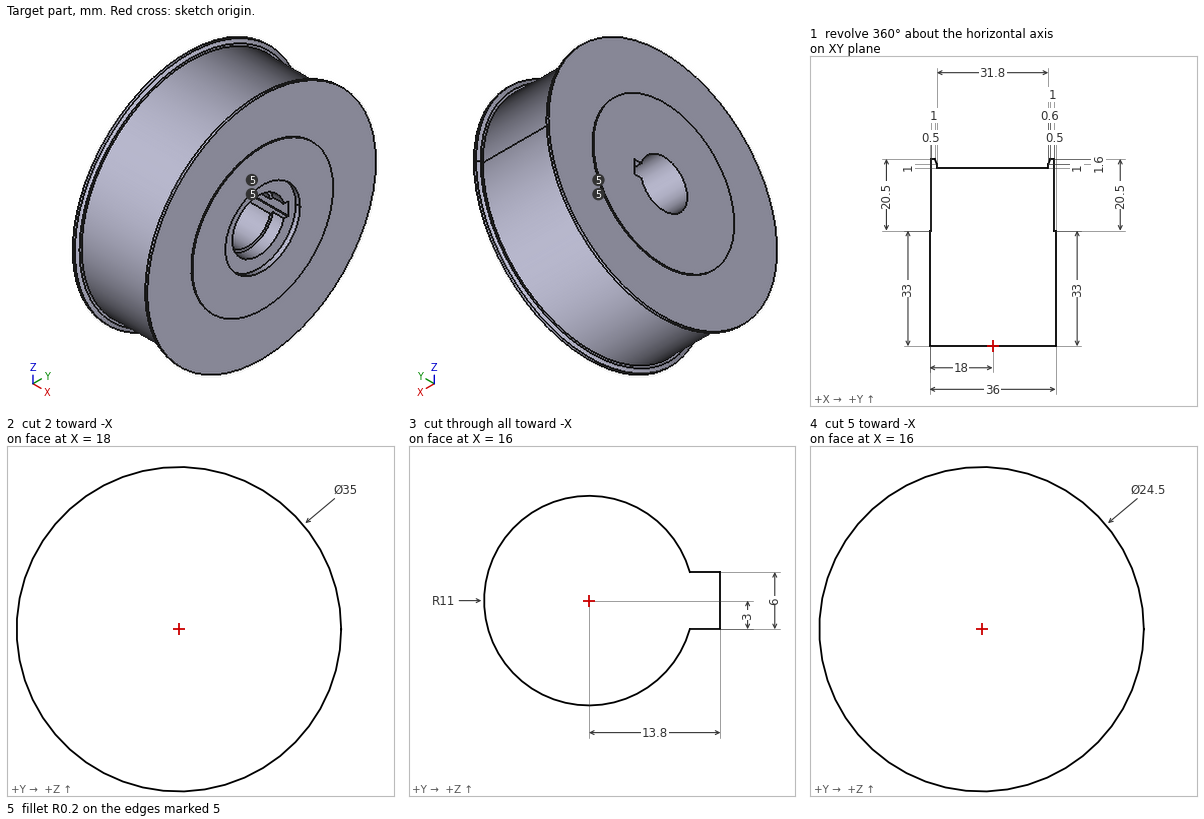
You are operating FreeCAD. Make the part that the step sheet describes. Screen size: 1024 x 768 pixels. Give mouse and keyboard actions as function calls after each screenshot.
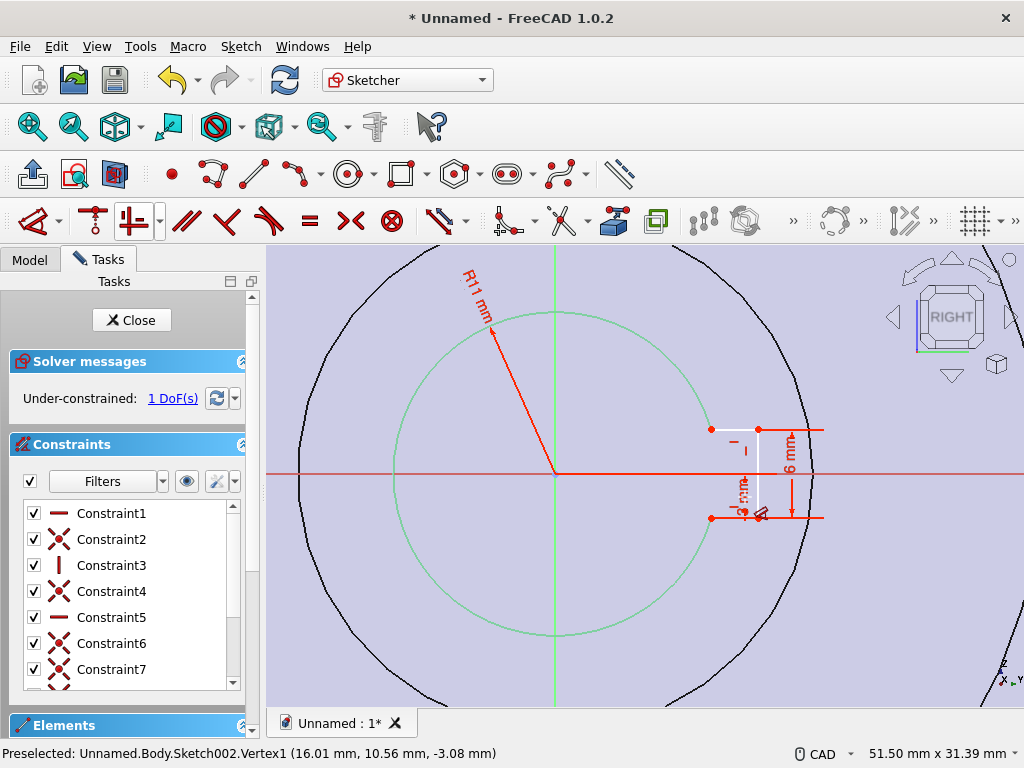
click(758, 518)
click(657, 552)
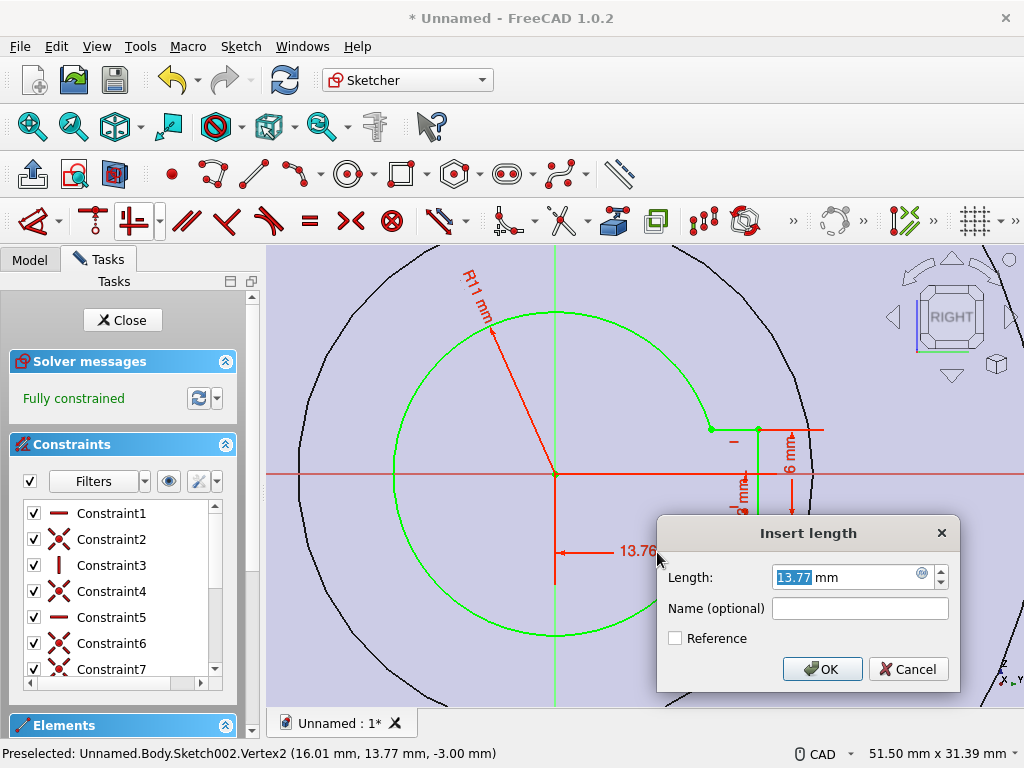
text(13.8)
key(Return)
key(Escape)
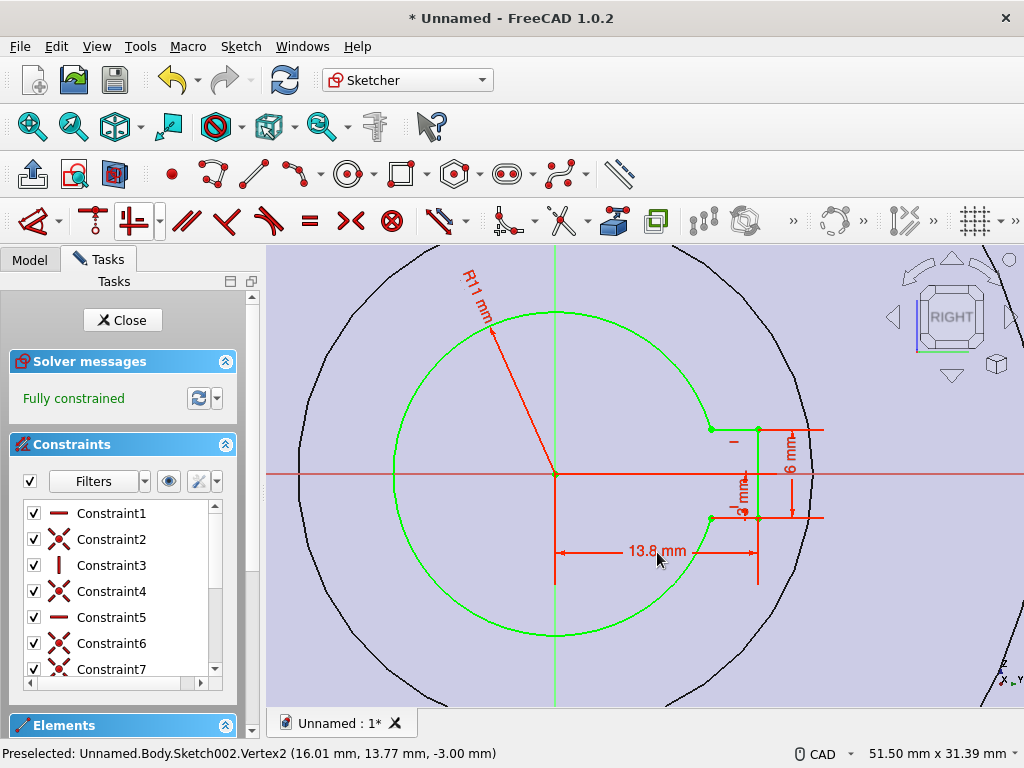
click(123, 320)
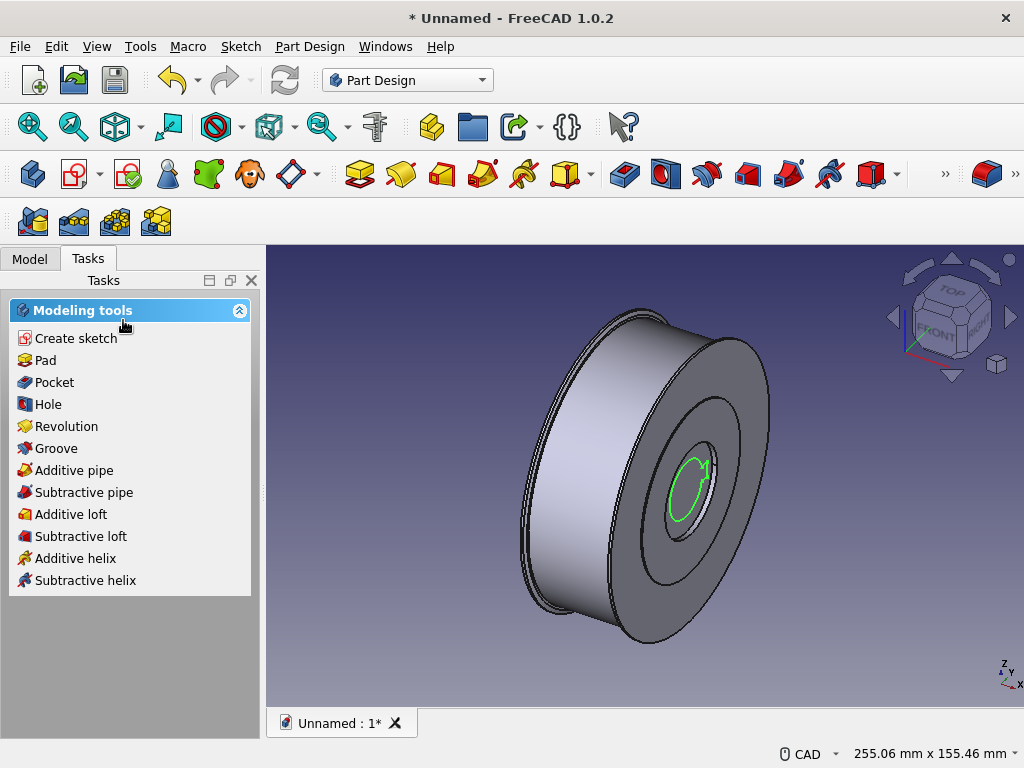
click(625, 174)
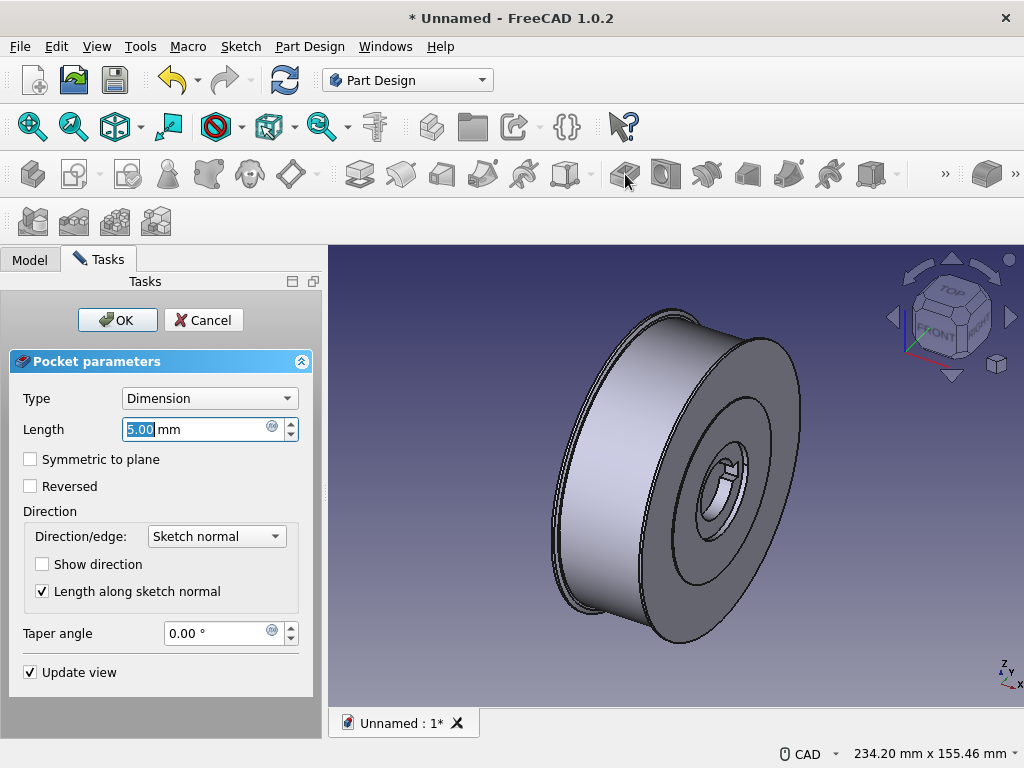
click(210, 398)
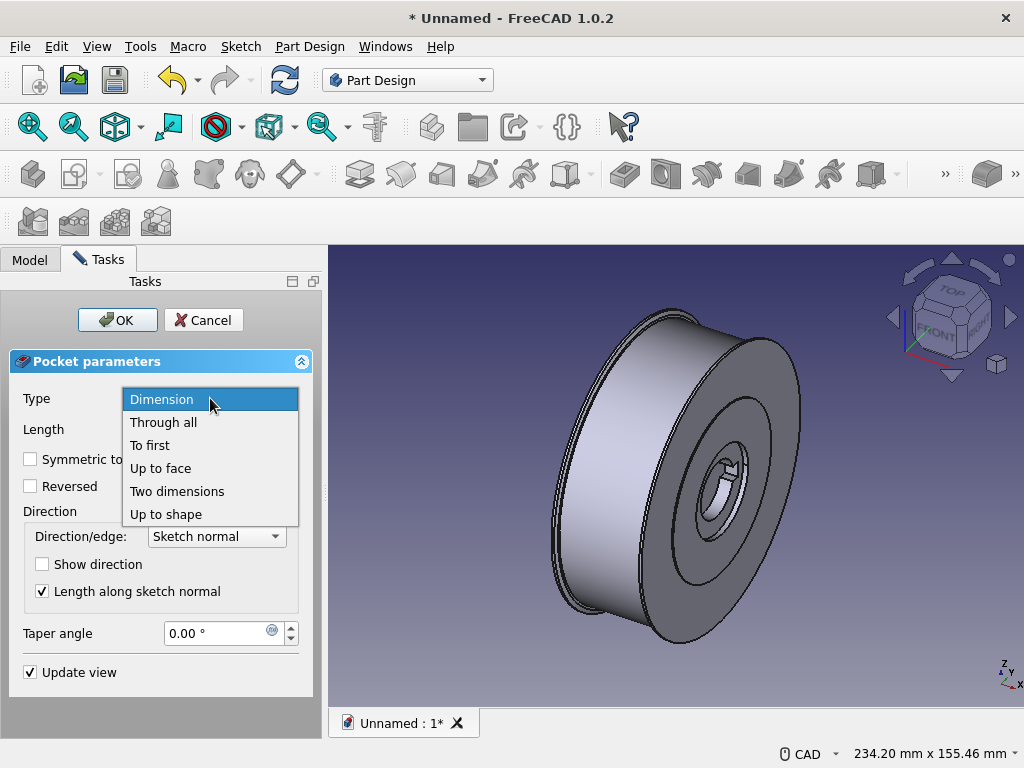
click(208, 422)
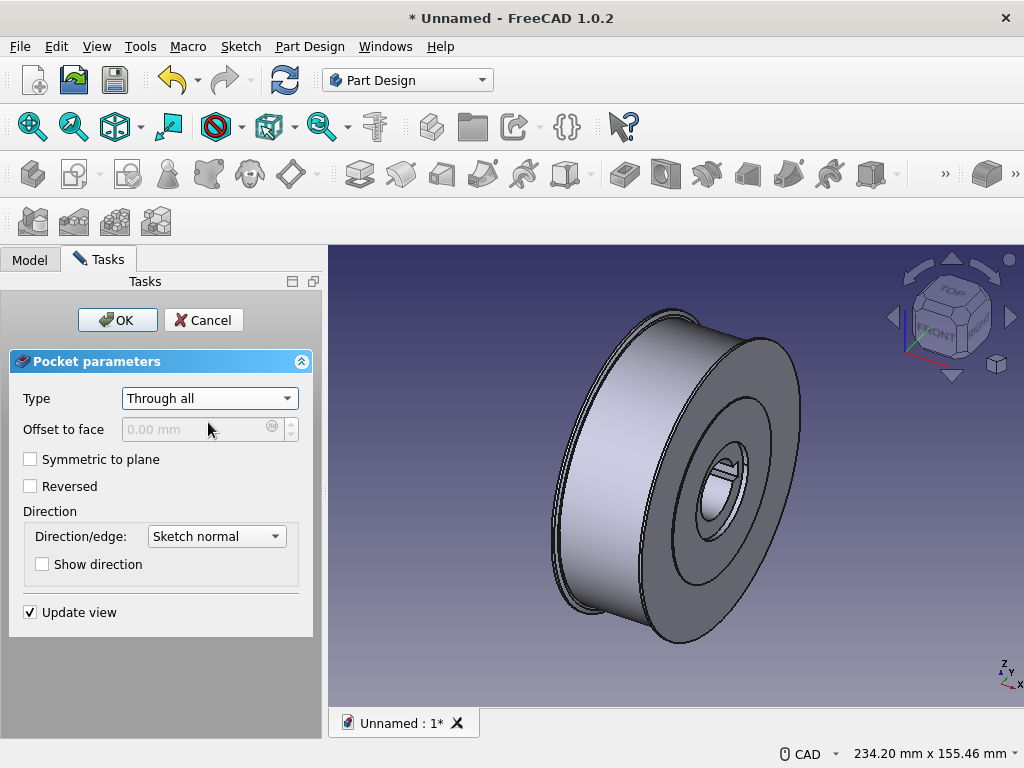
click(118, 320)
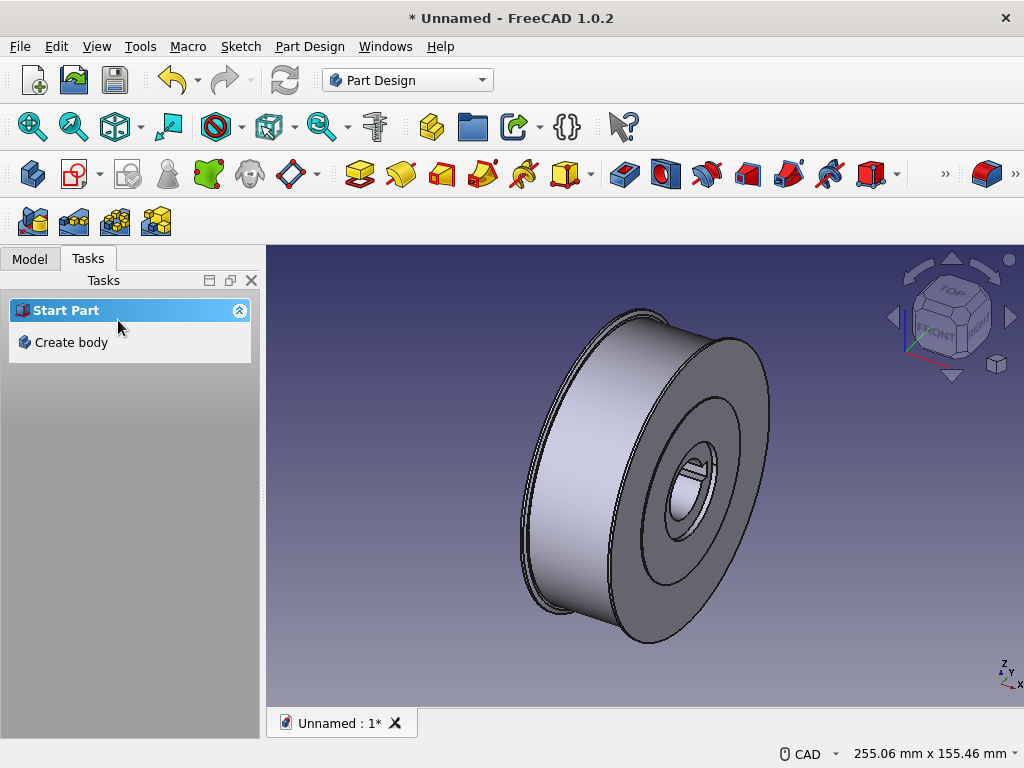
key(0)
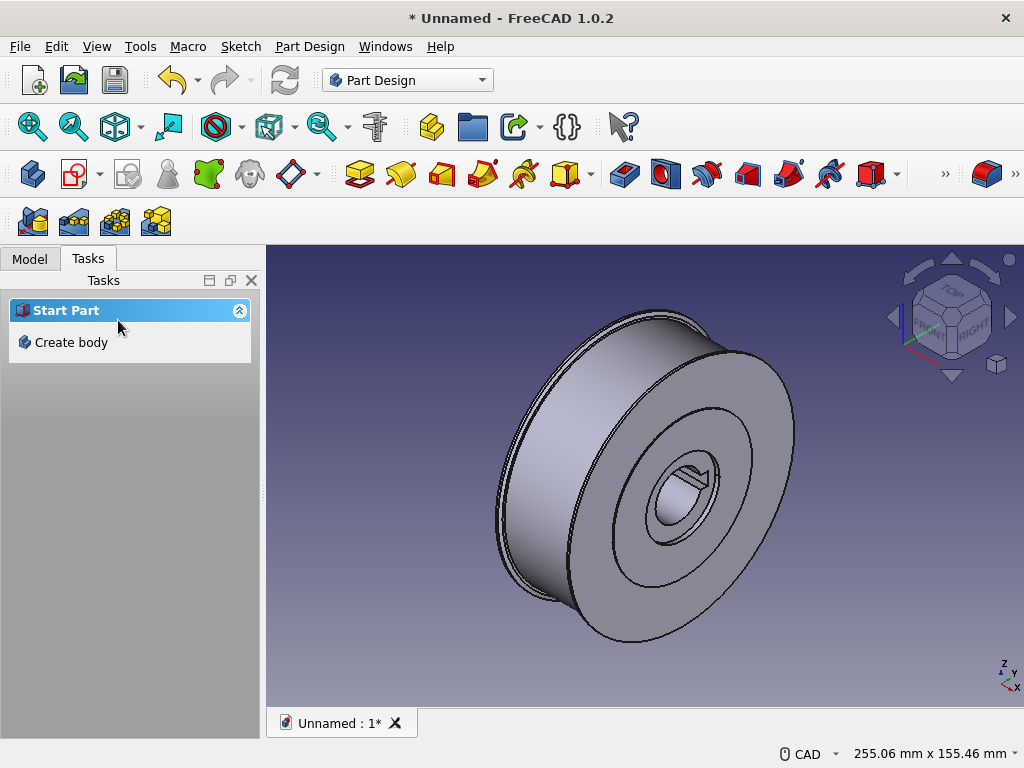
click(700, 458)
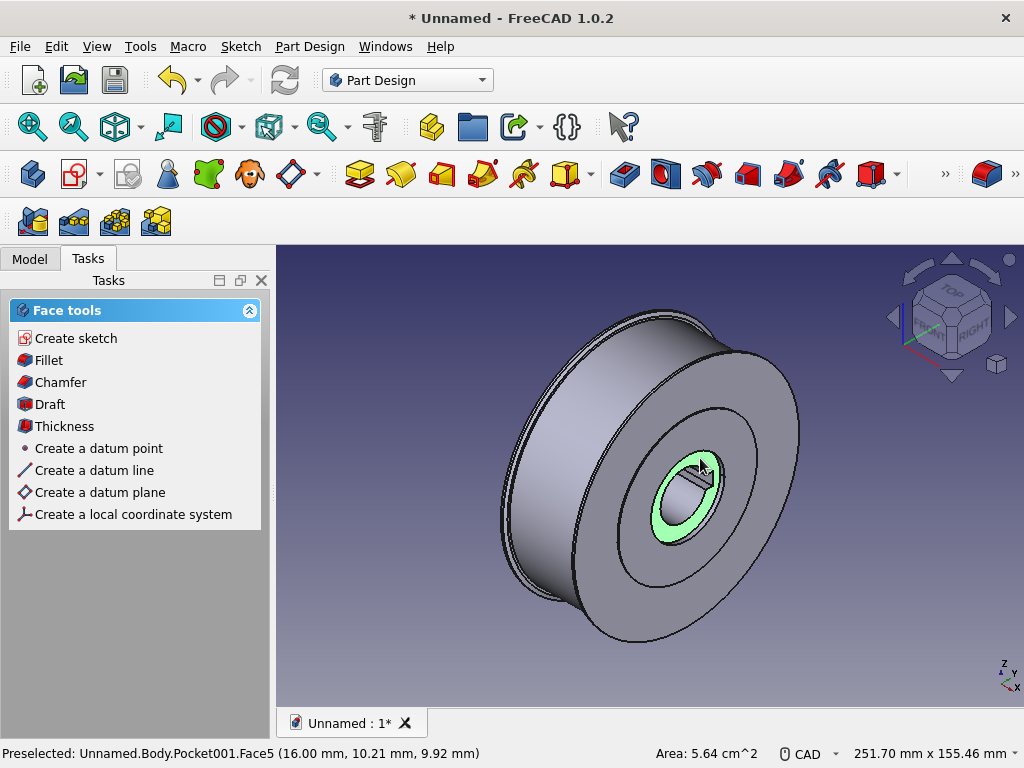
click(74, 174)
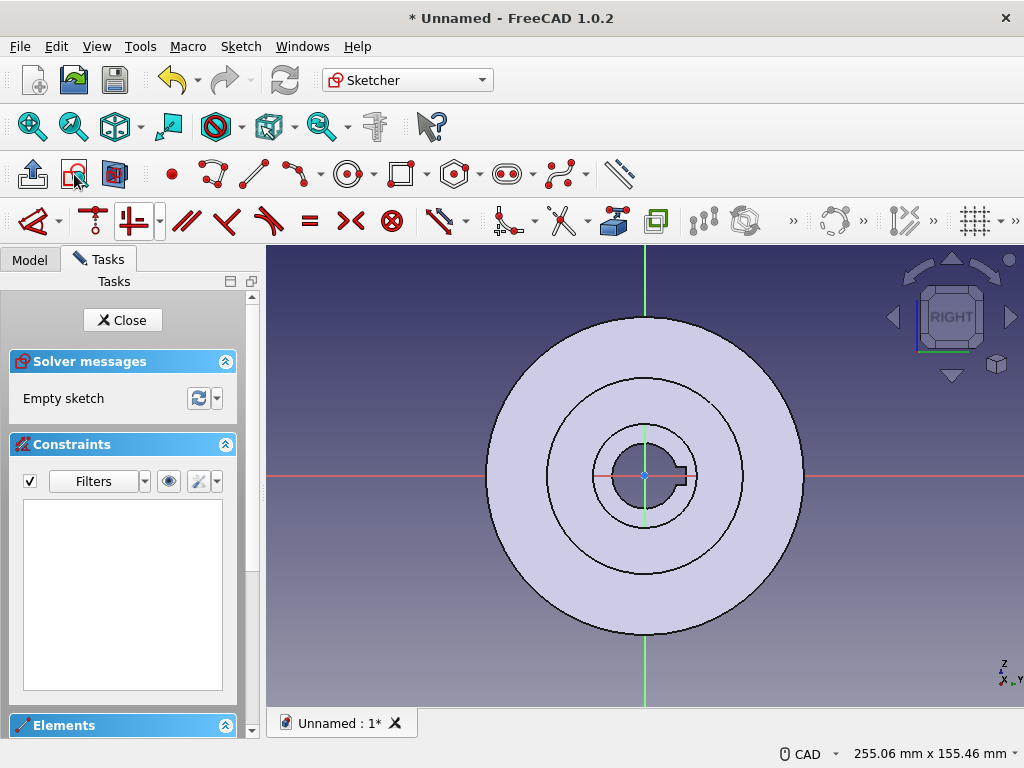
scroll(667, 476, up, 7)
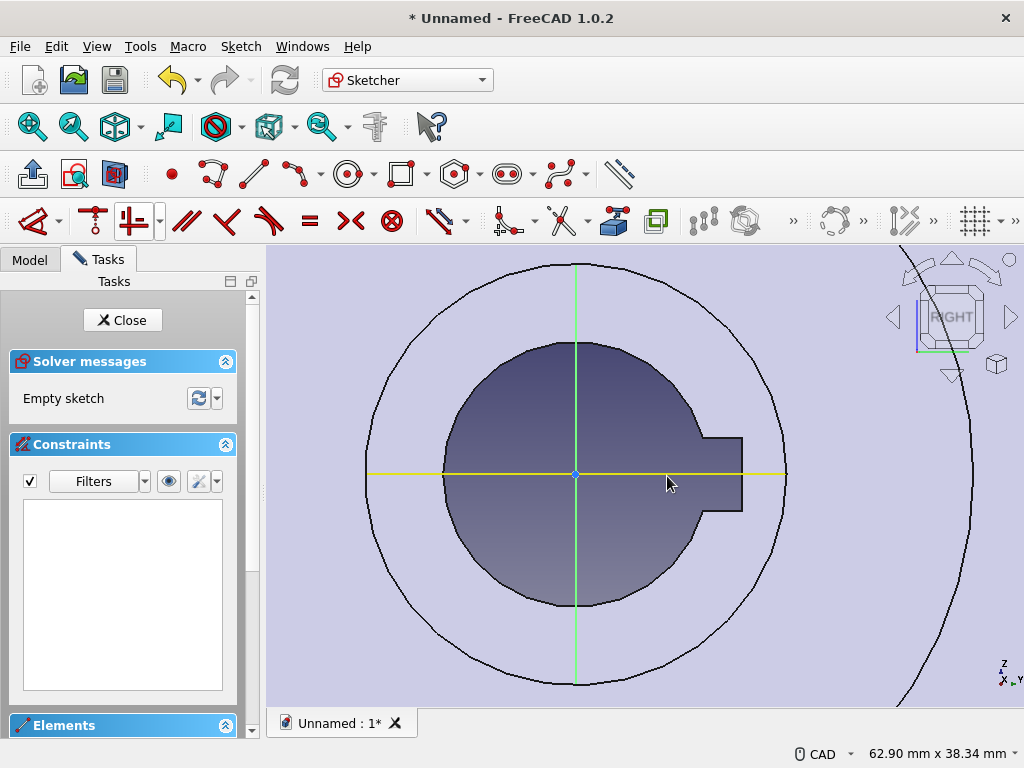
click(348, 174)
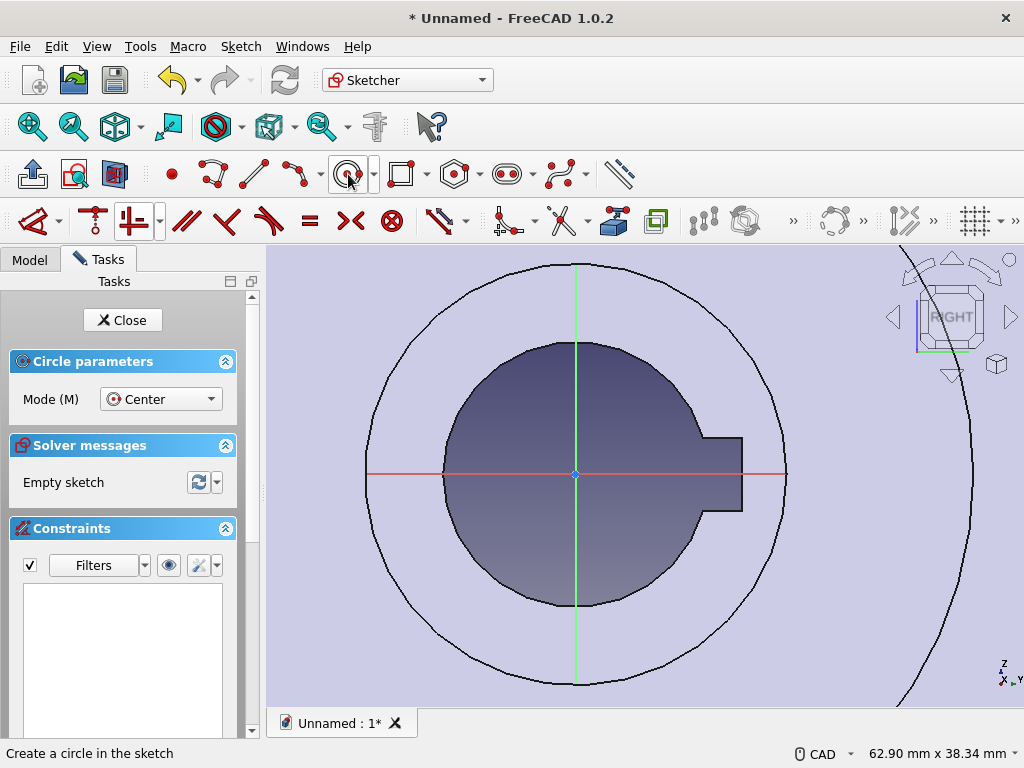
click(576, 474)
click(680, 370)
key(Escape)